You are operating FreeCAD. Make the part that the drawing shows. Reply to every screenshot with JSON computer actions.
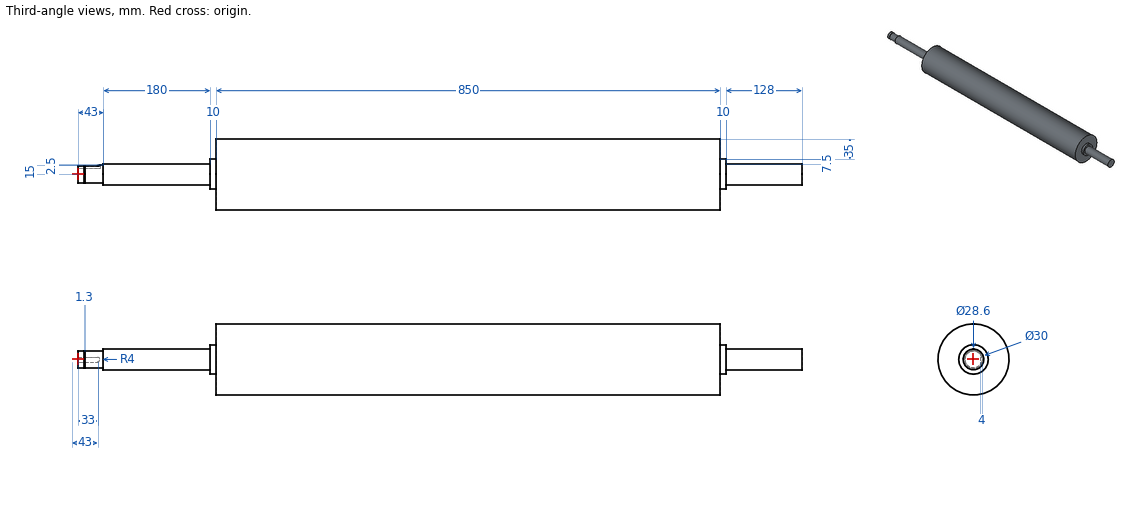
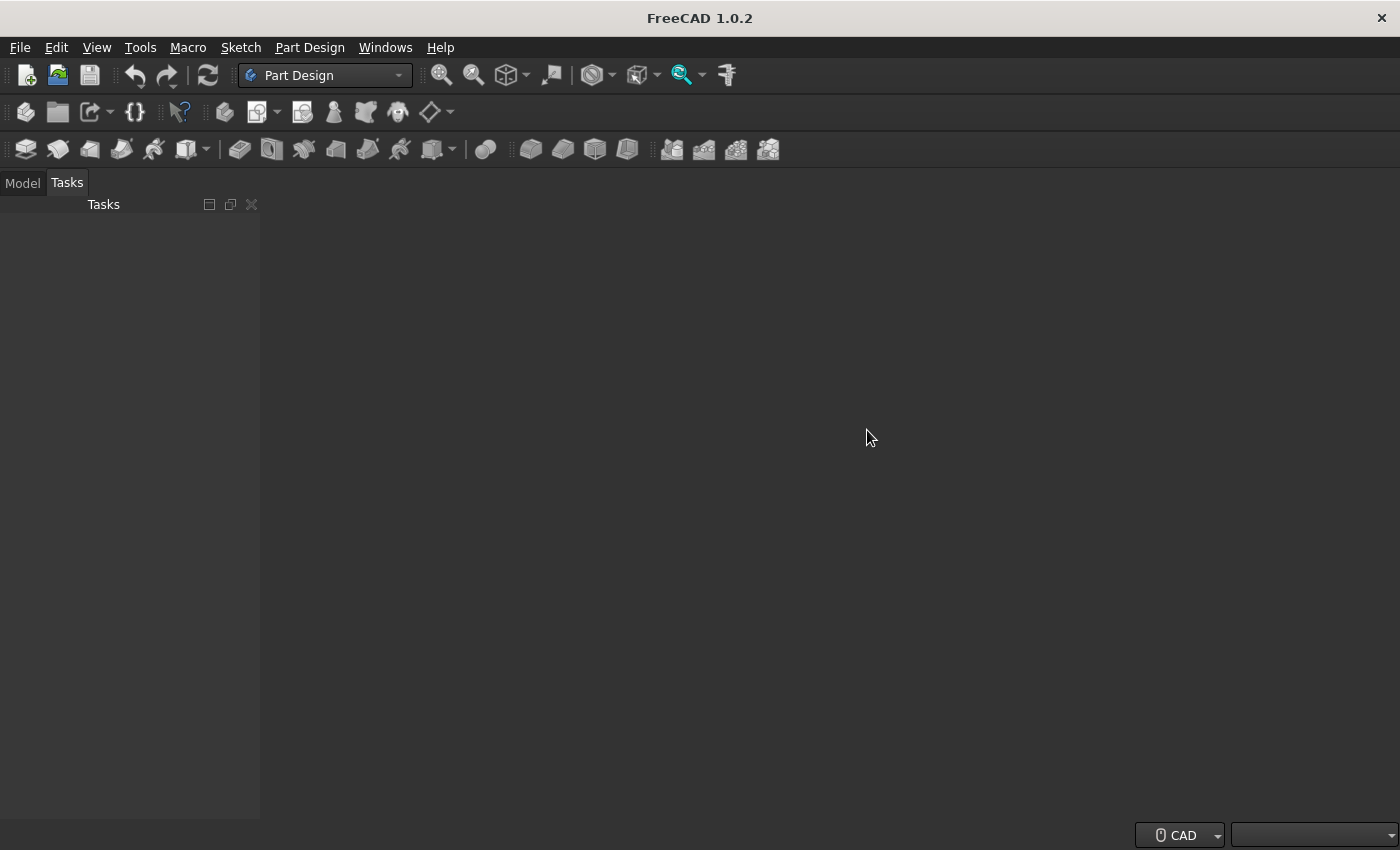
{"action": "left_click", "coordinate": [26, 76]}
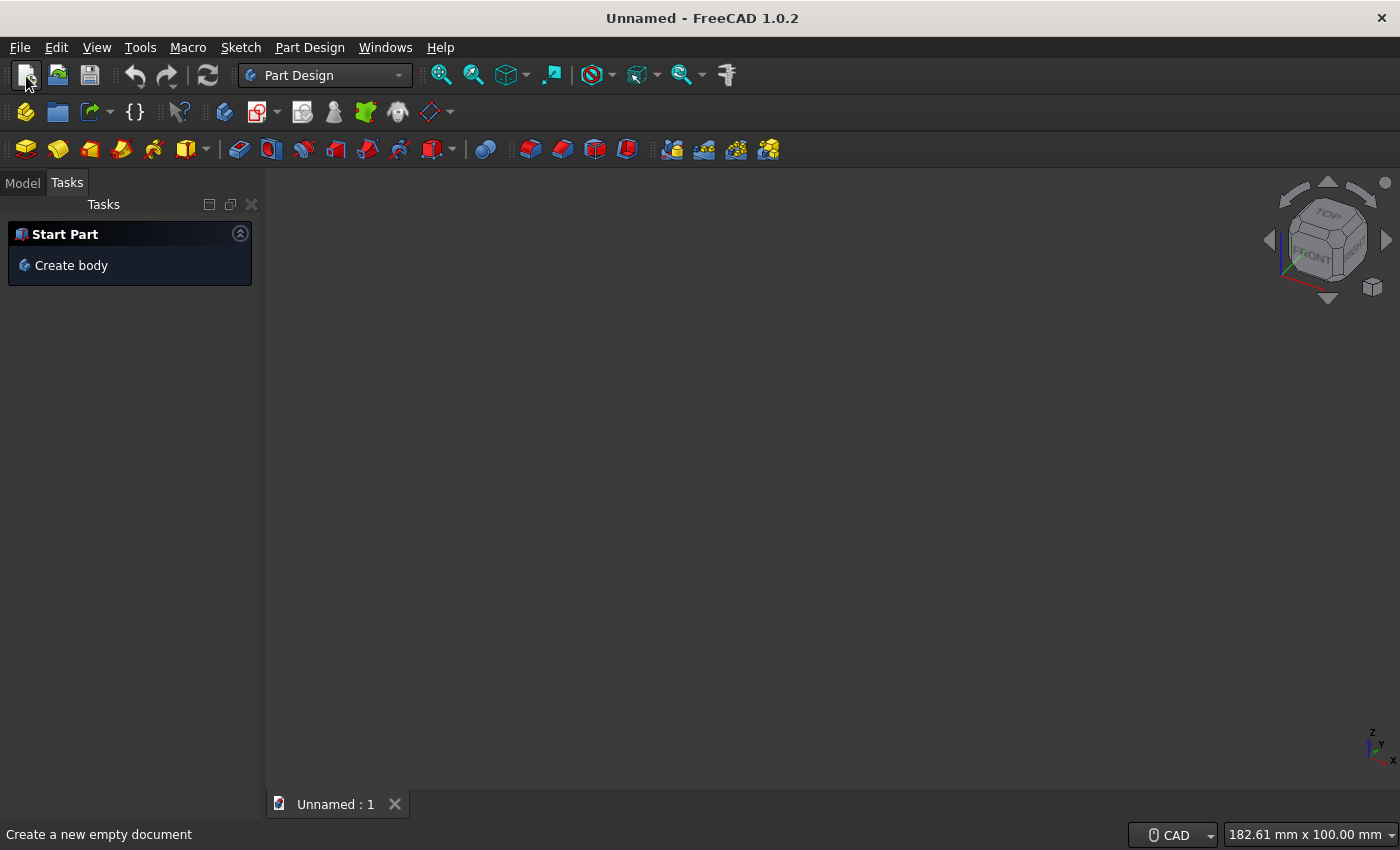
{"action": "left_click", "coordinate": [258, 112]}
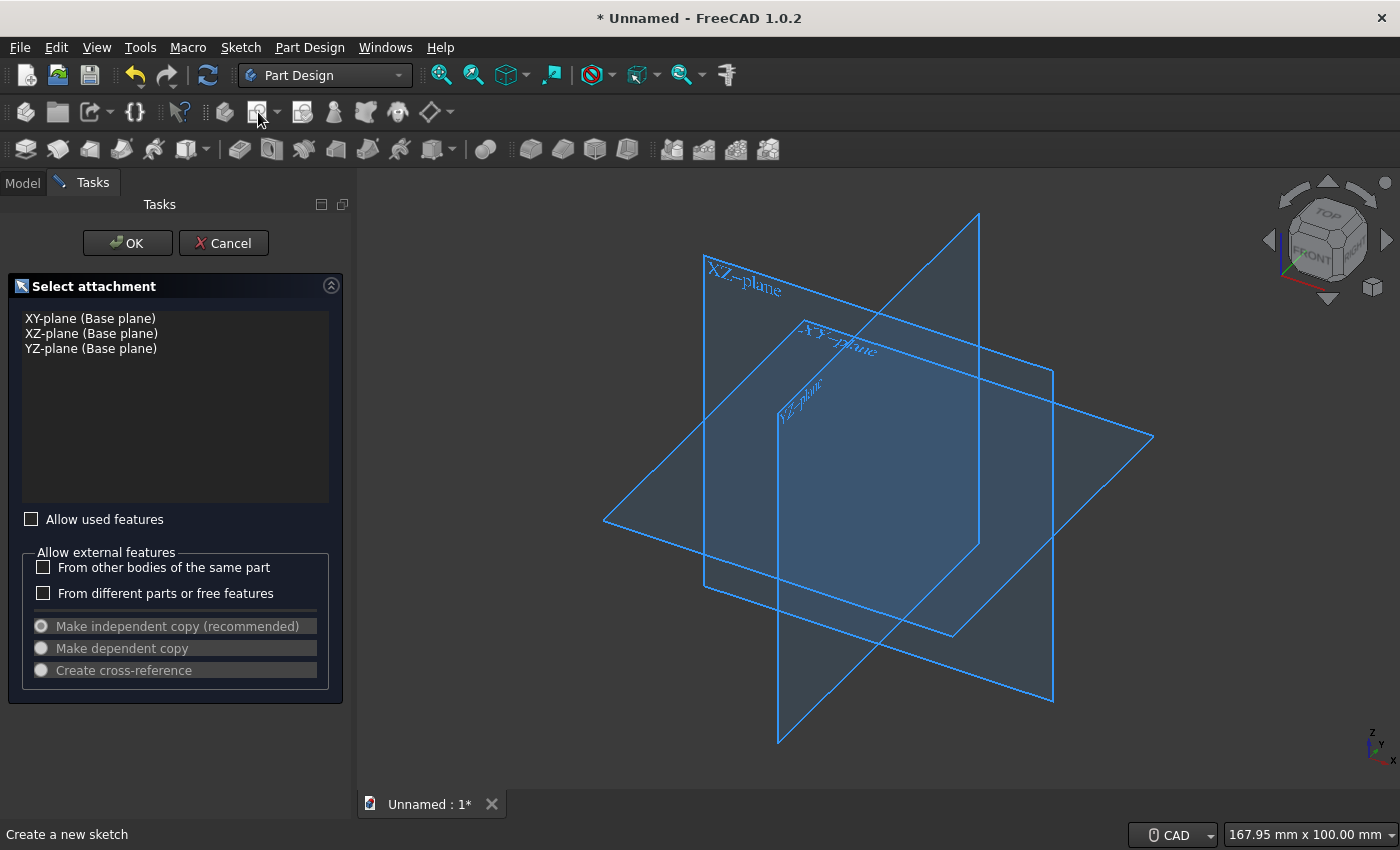
{"action": "left_click", "coordinate": [82, 318]}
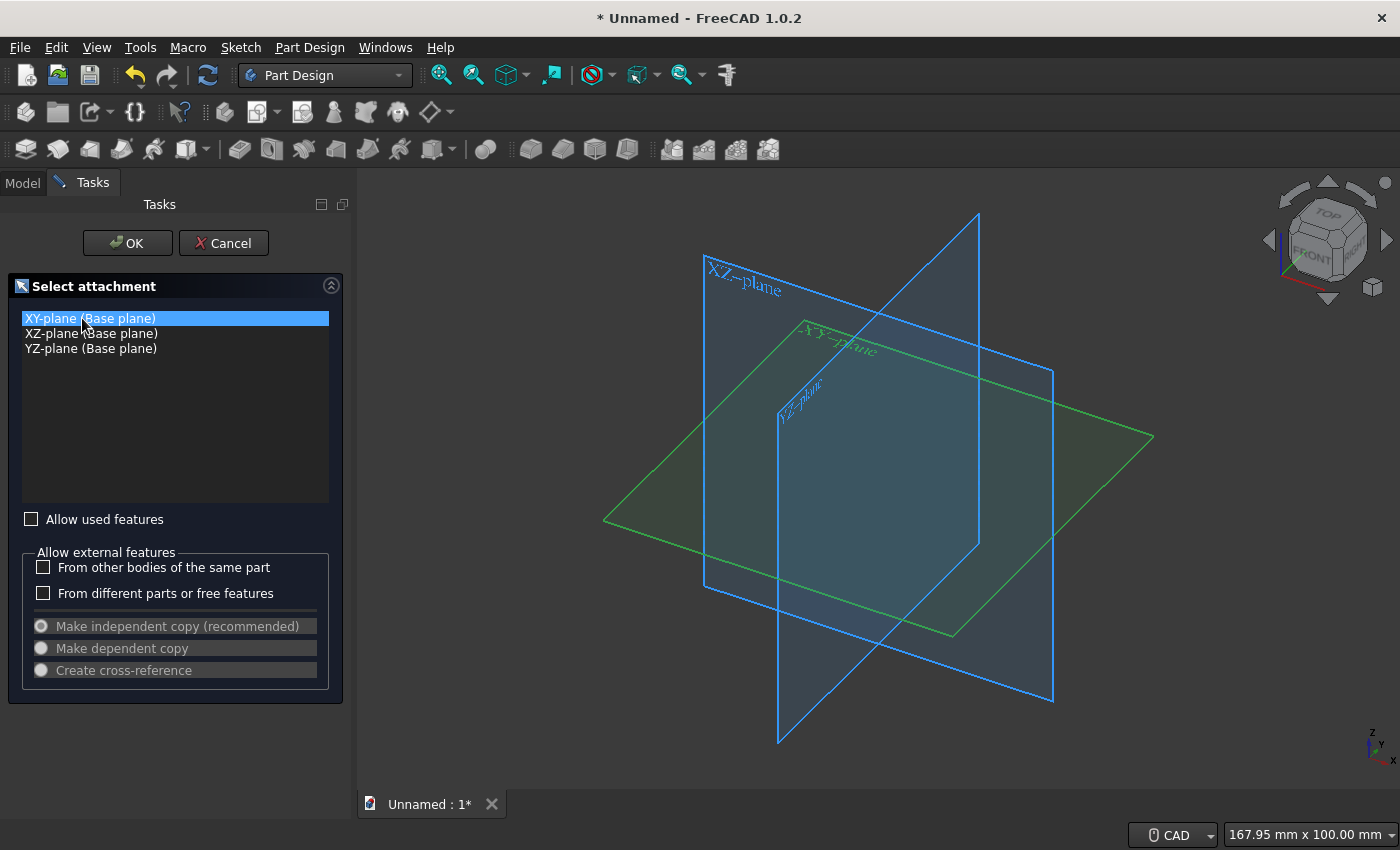
{"action": "left_click", "coordinate": [128, 243]}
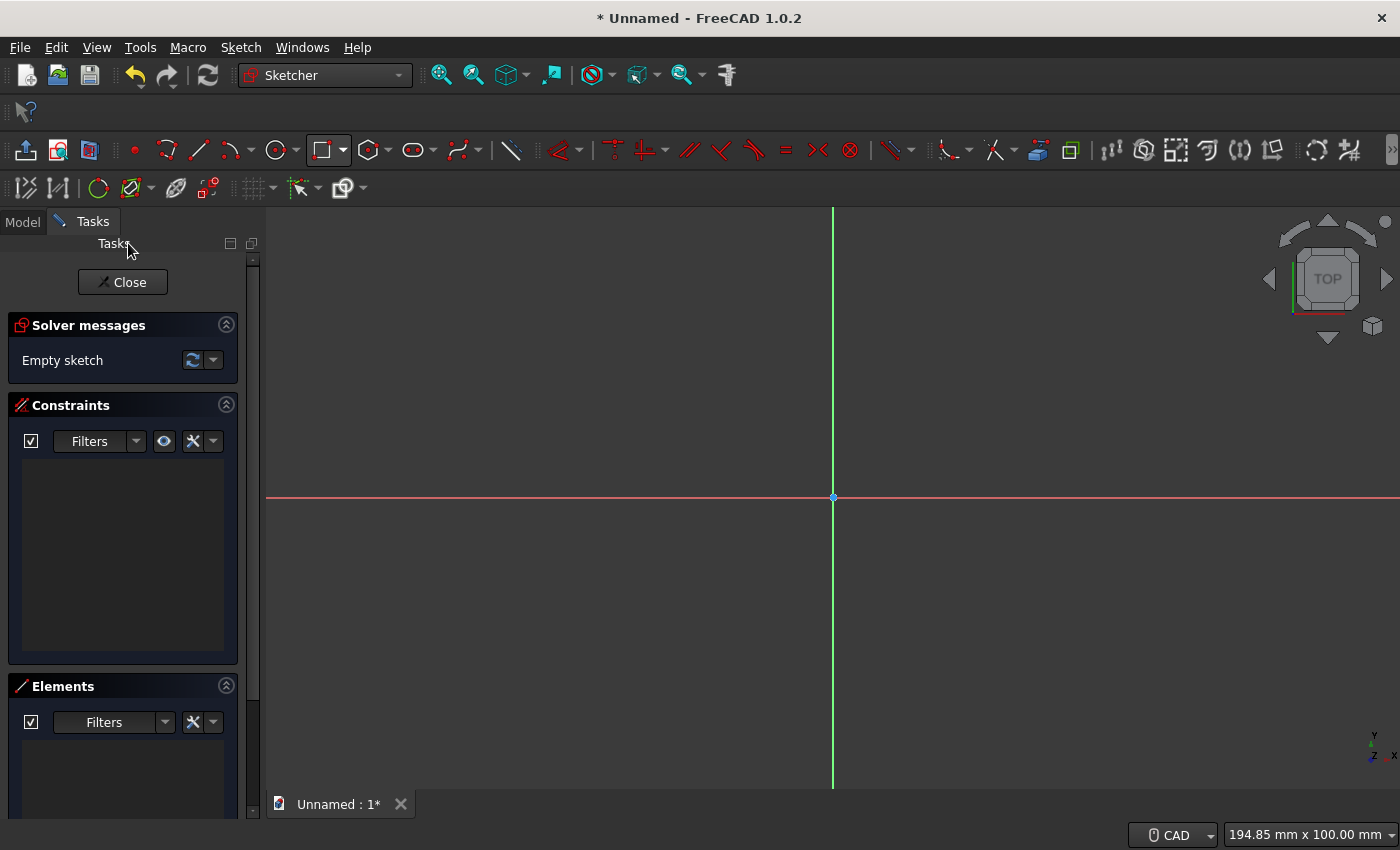
{"action": "scroll", "coordinate": [403, 515], "scroll_direction": "down", "scroll_amount": 12}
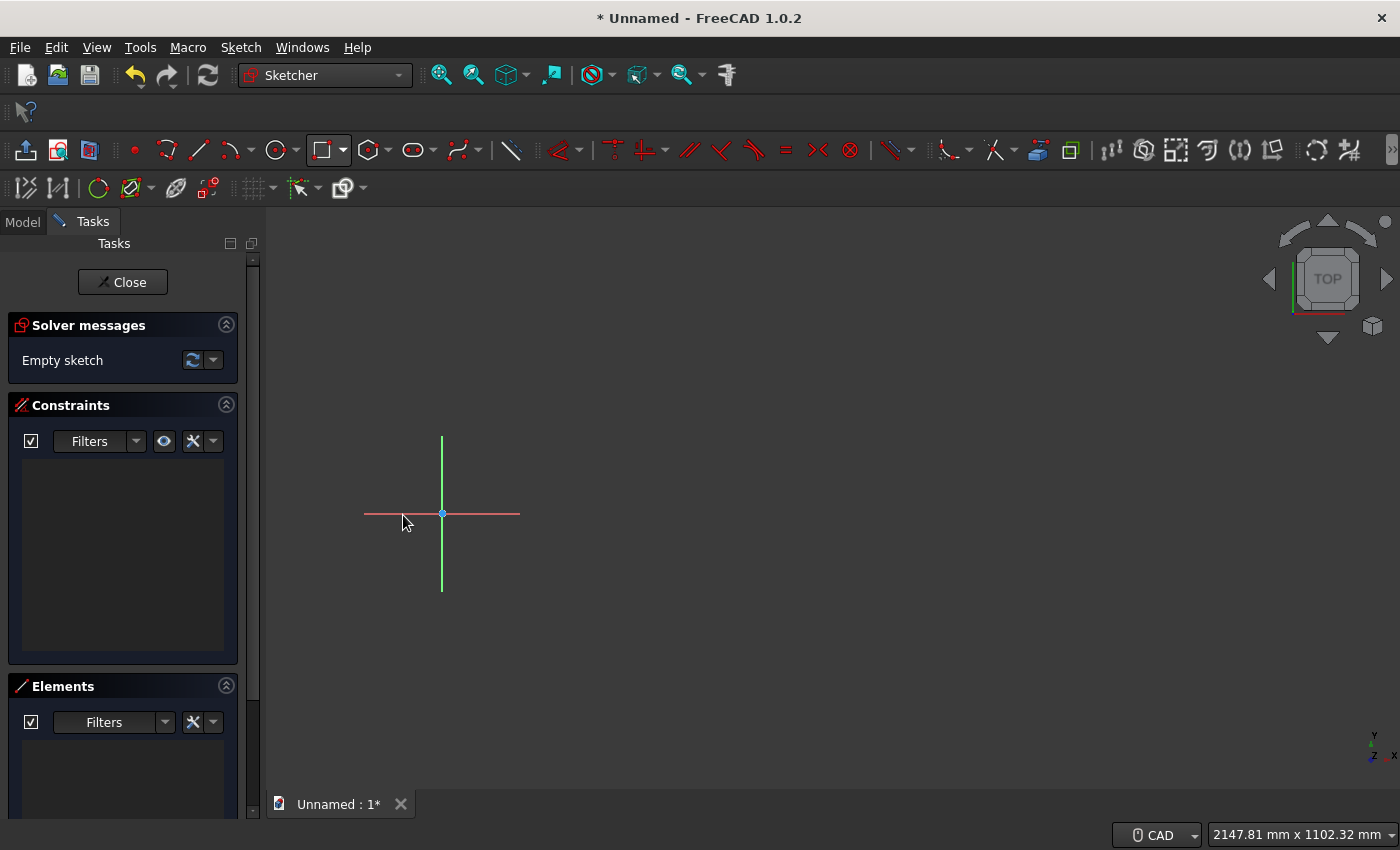
{"action": "key", "text": "g m"}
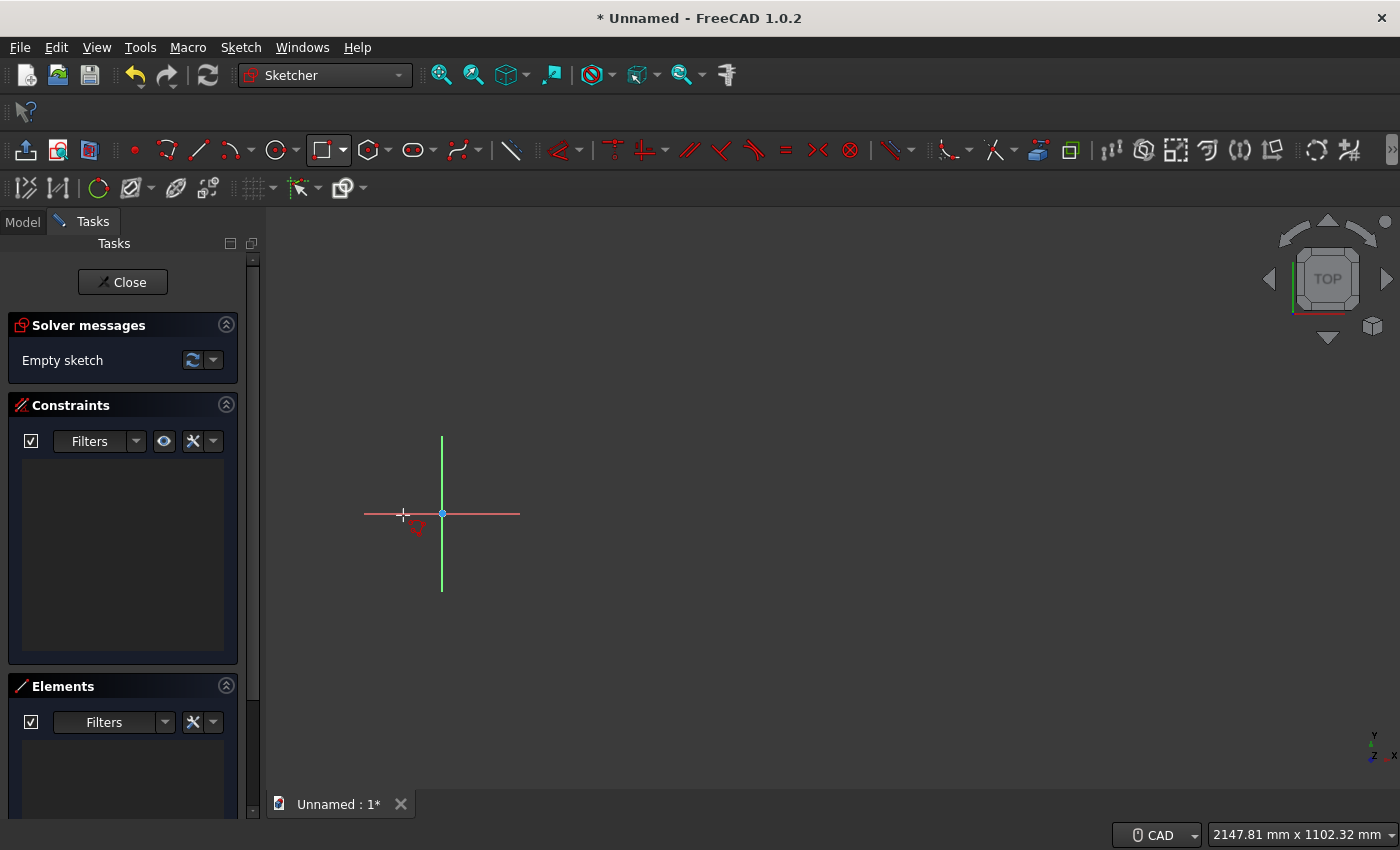
{"action": "left_click", "coordinate": [442, 514]}
{"action": "left_click", "coordinate": [1087, 505]}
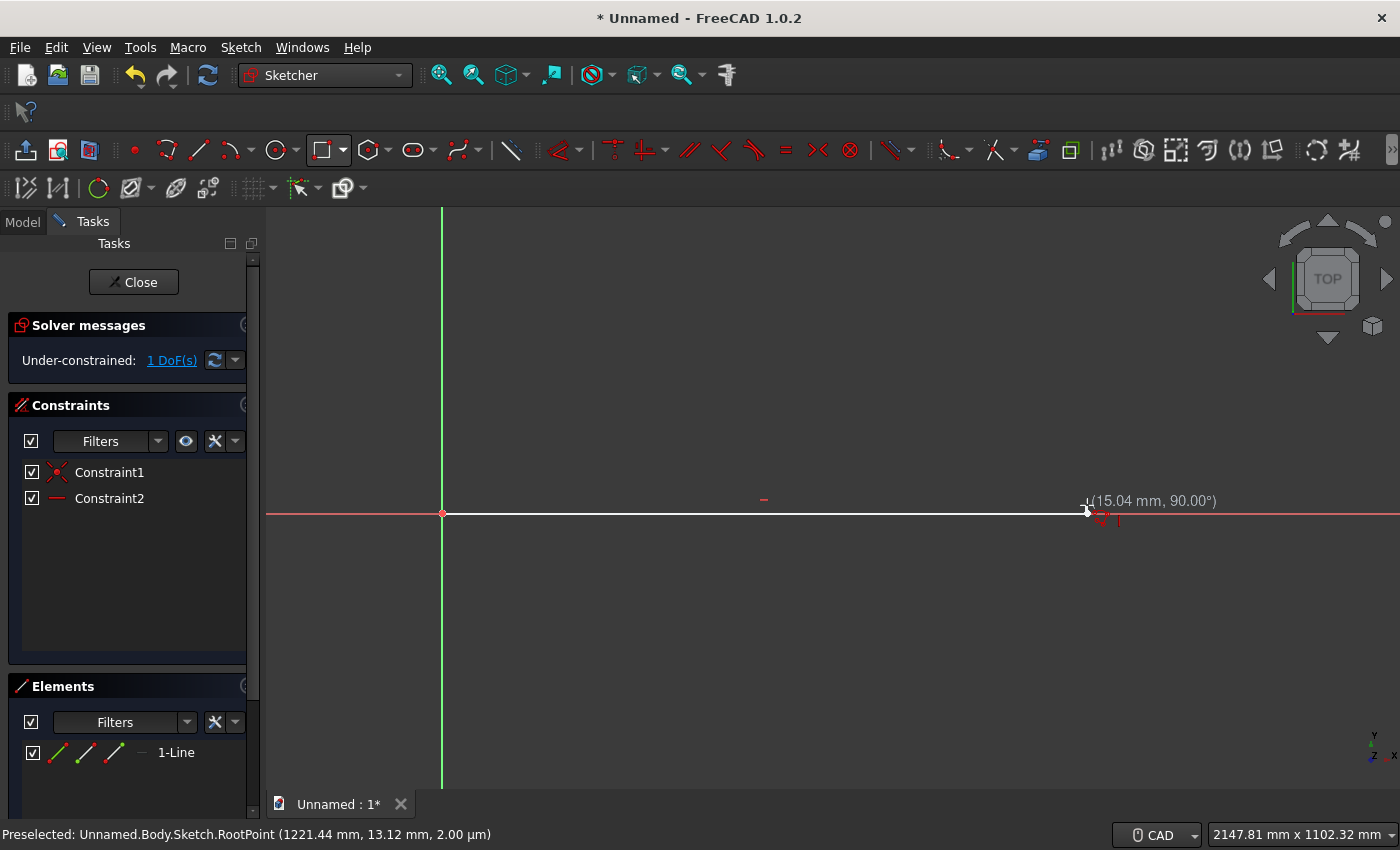
{"action": "scroll", "coordinate": [1087, 505], "scroll_direction": "up", "scroll_amount": 3}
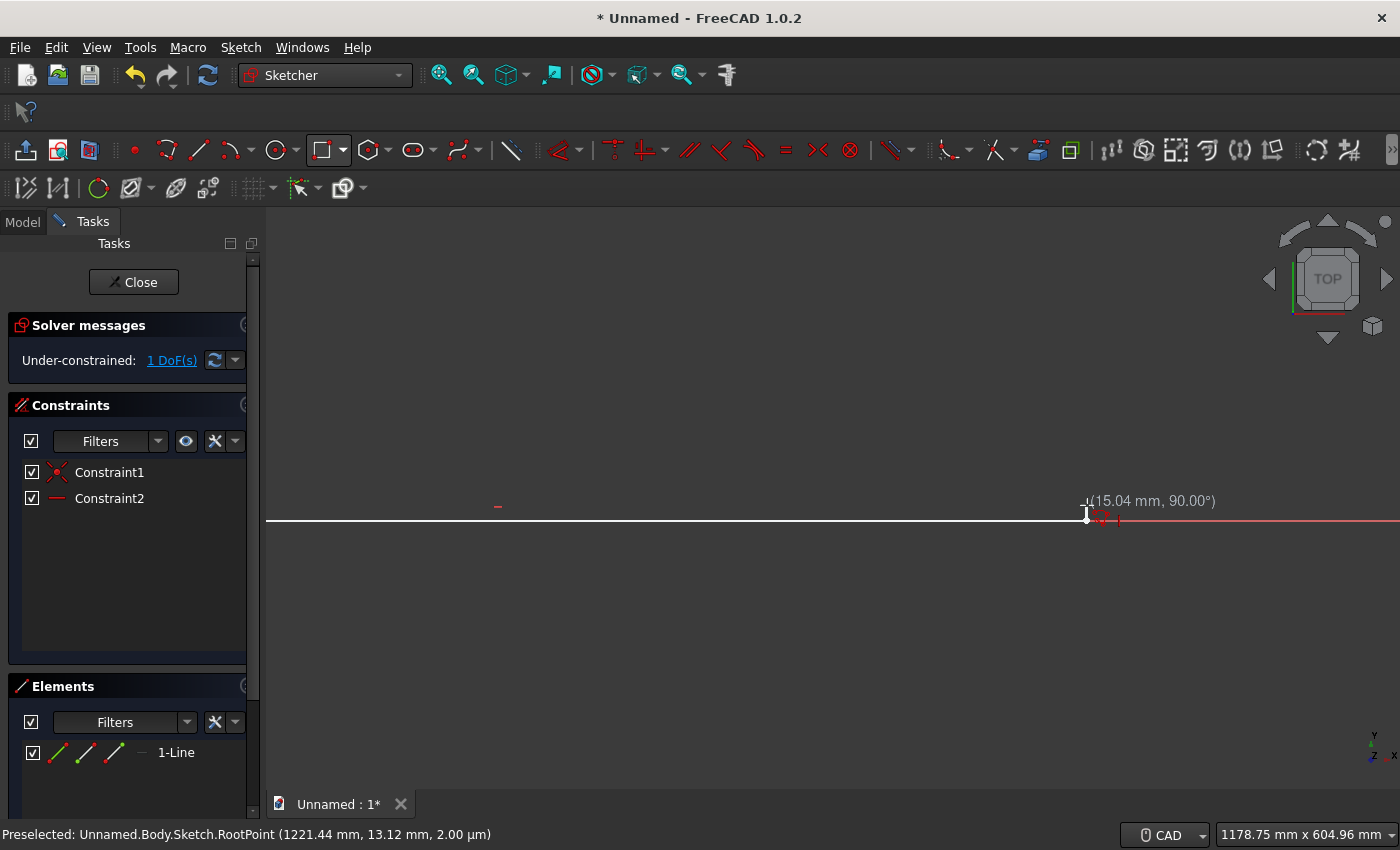
{"action": "left_click", "coordinate": [1086, 504]}
{"action": "left_click", "coordinate": [963, 504]}